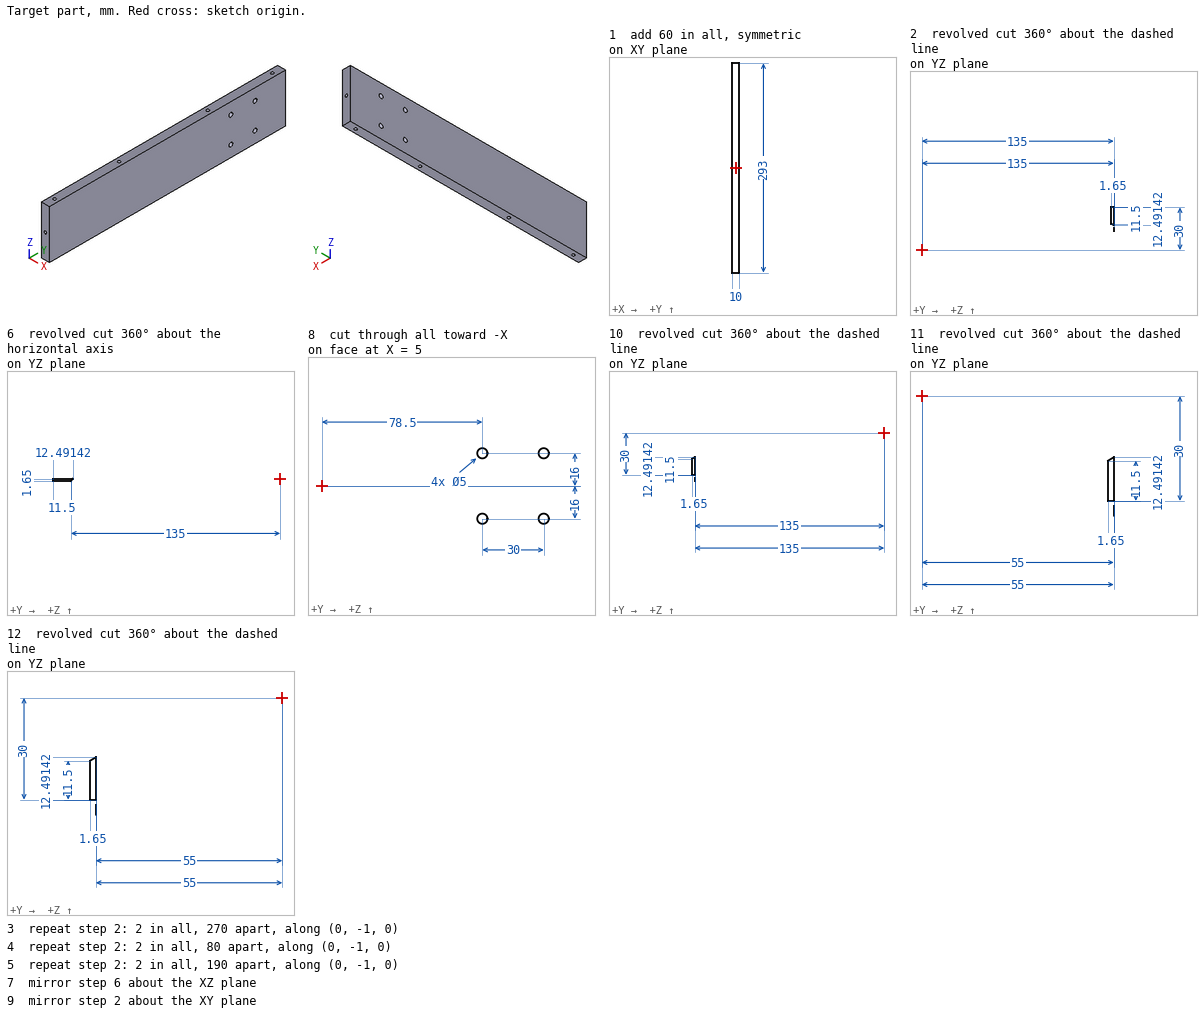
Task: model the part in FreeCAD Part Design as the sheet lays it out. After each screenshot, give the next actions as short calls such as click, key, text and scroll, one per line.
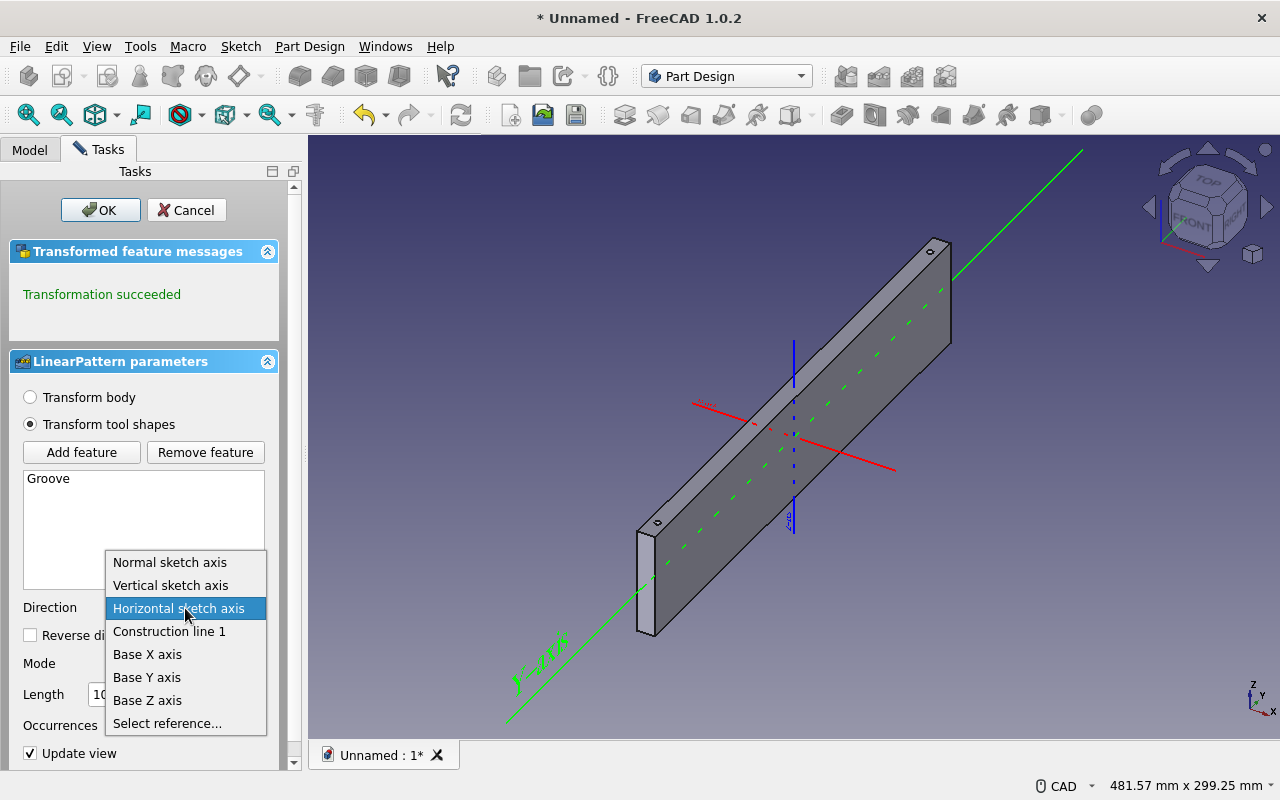
click(184, 678)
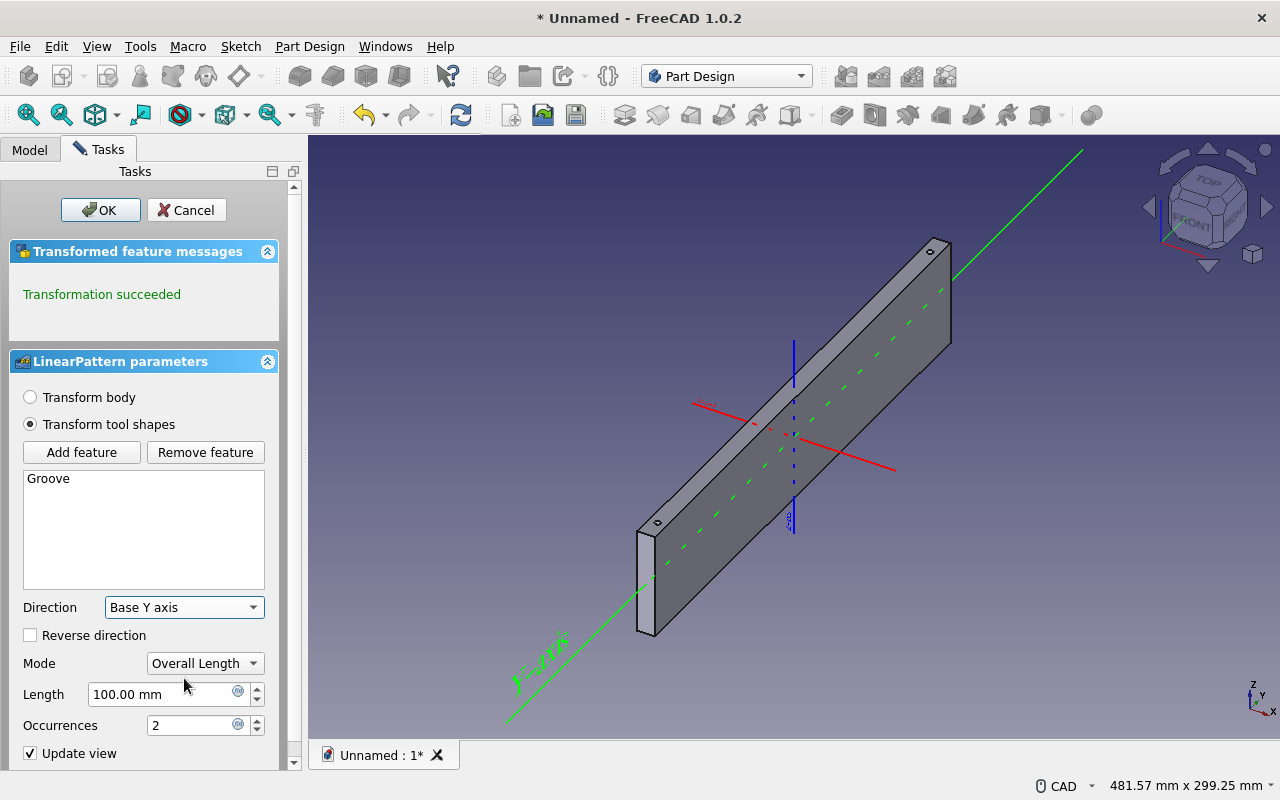
click(206, 664)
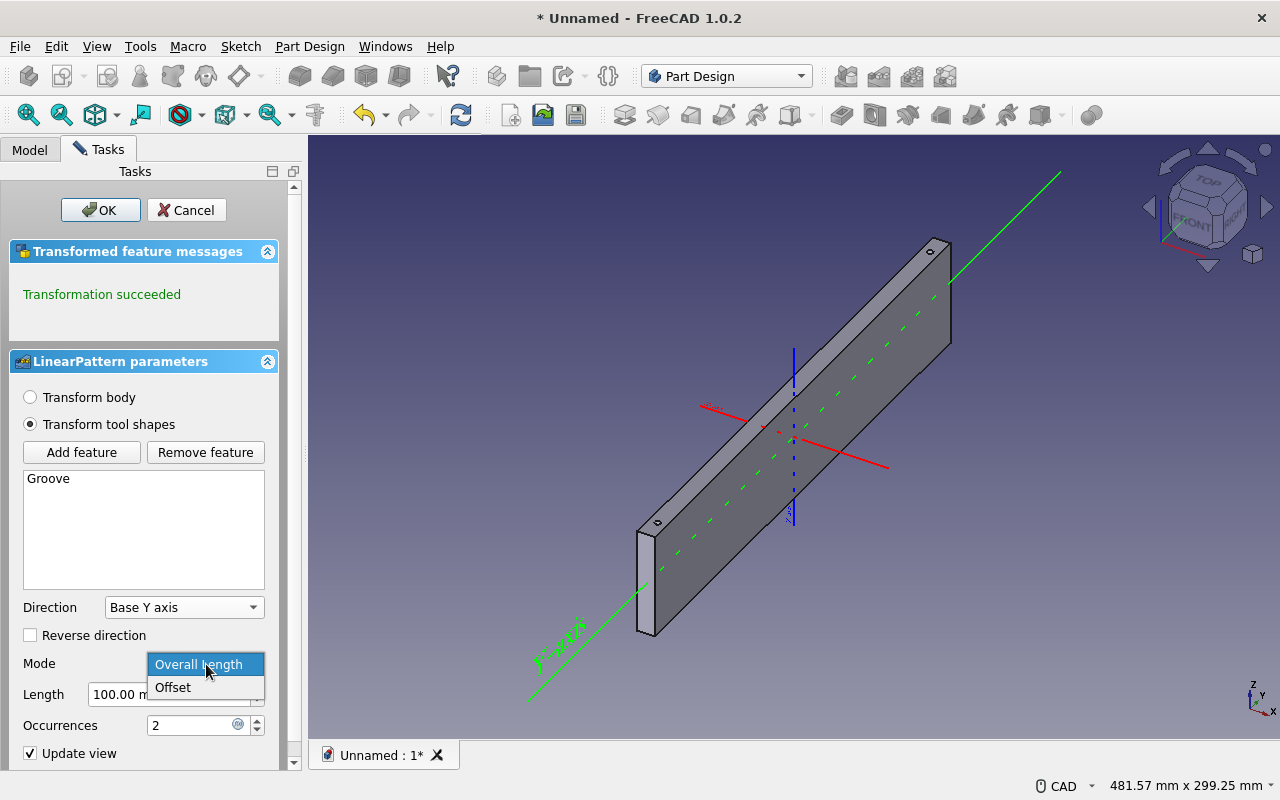
click(204, 688)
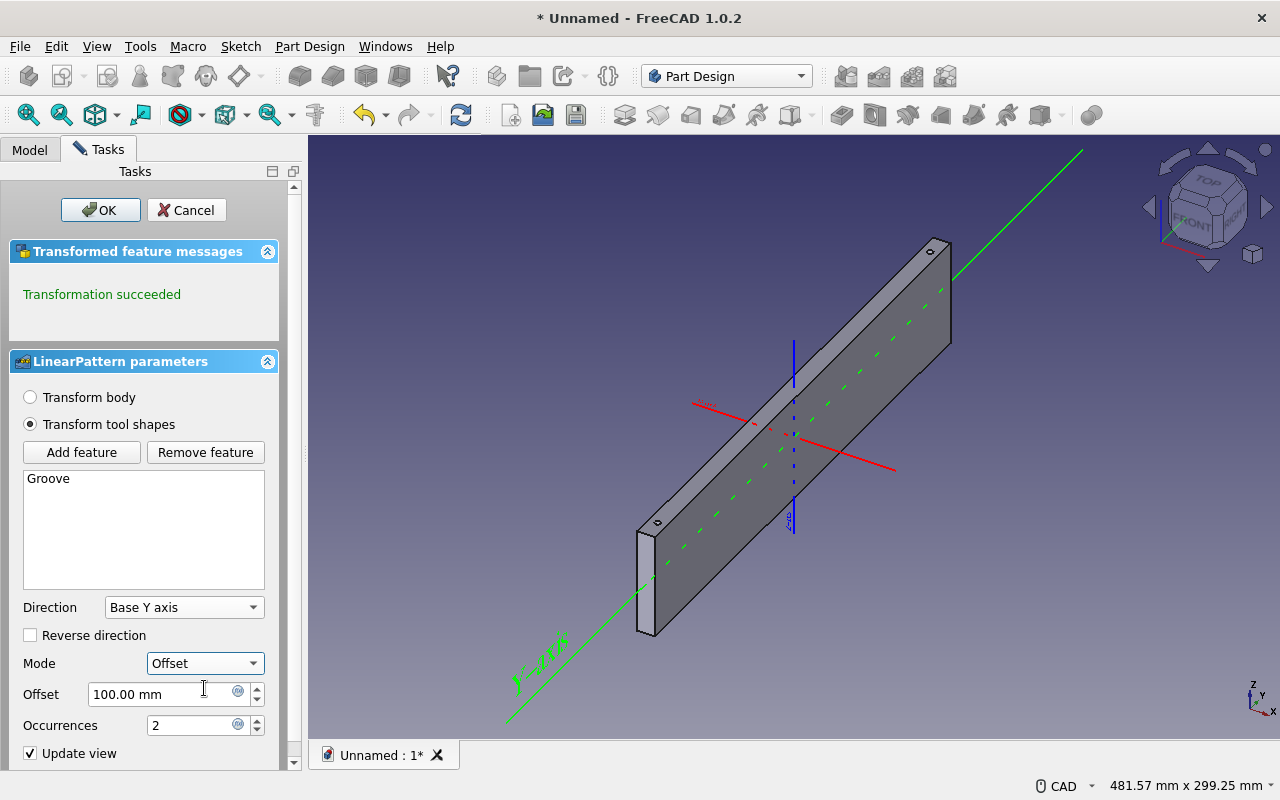
triple_click(170, 694)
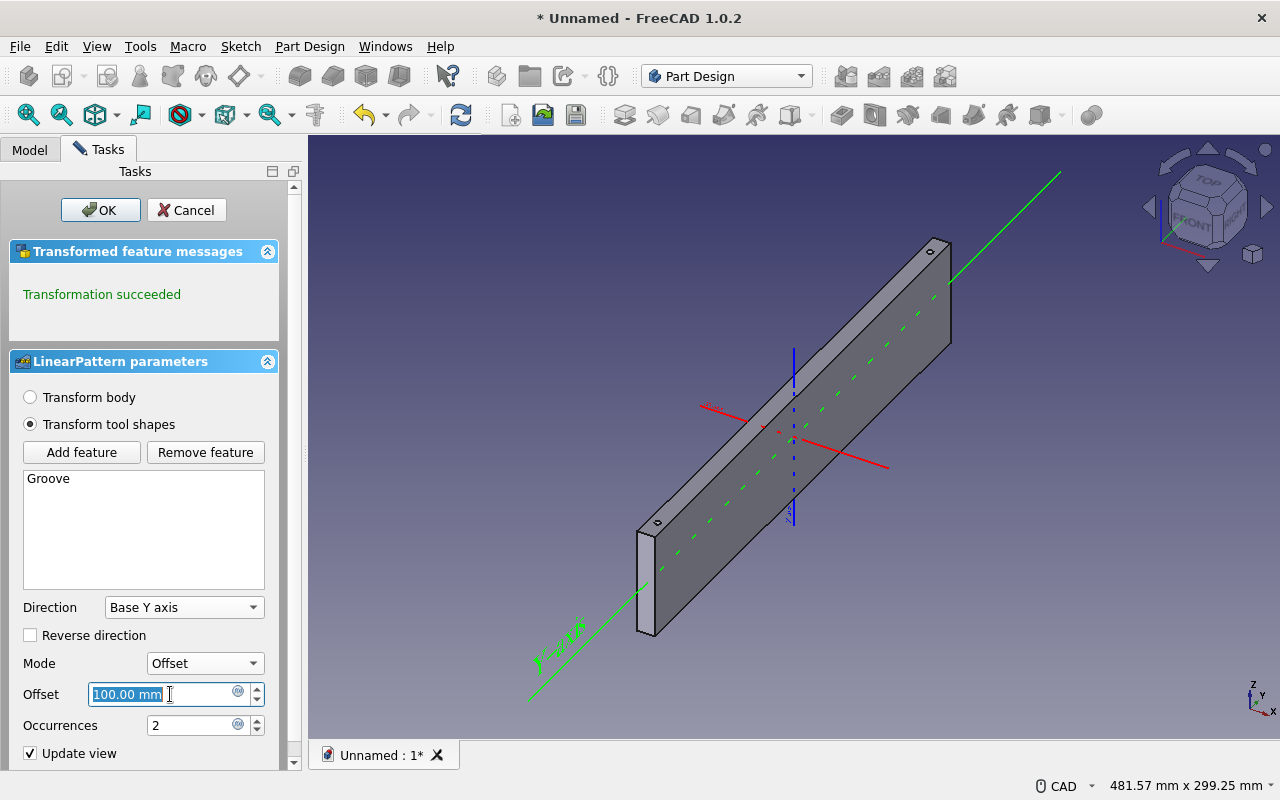
text(80)
key(Tab)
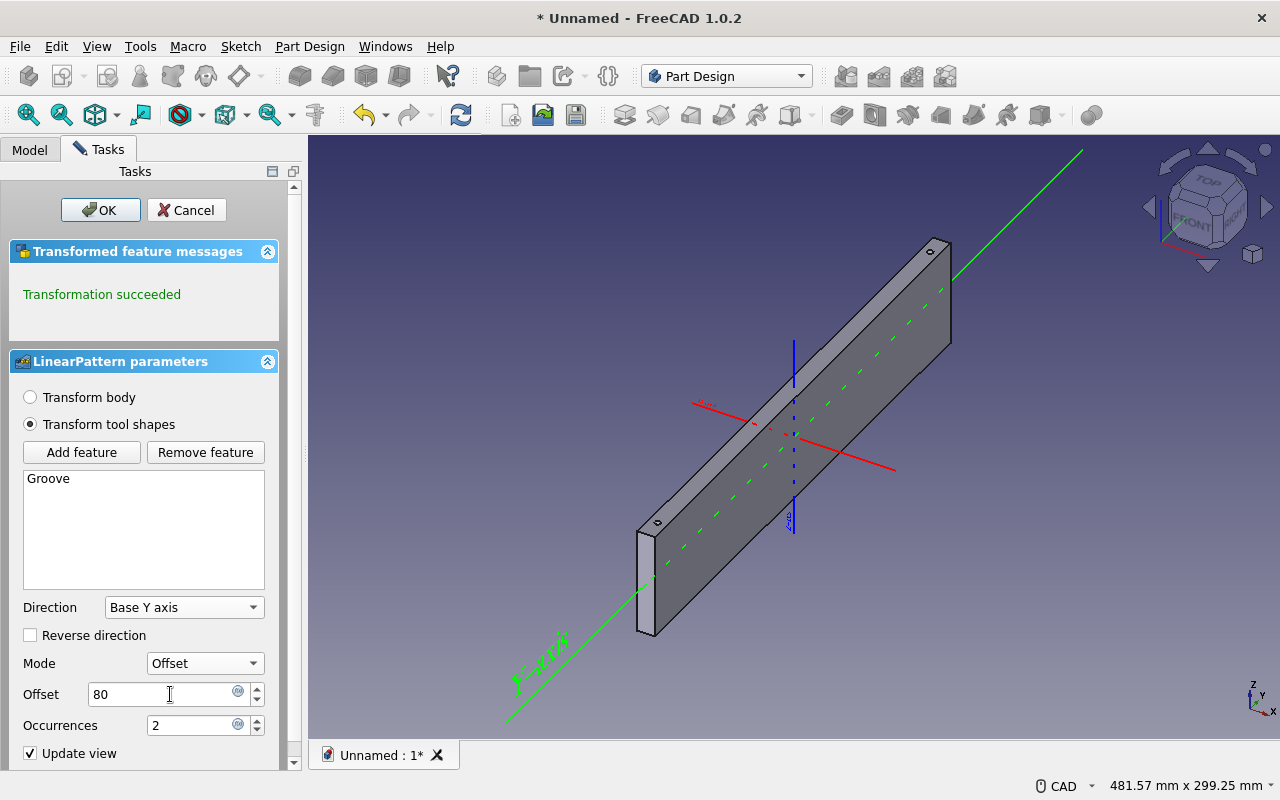
triple_click(199, 726)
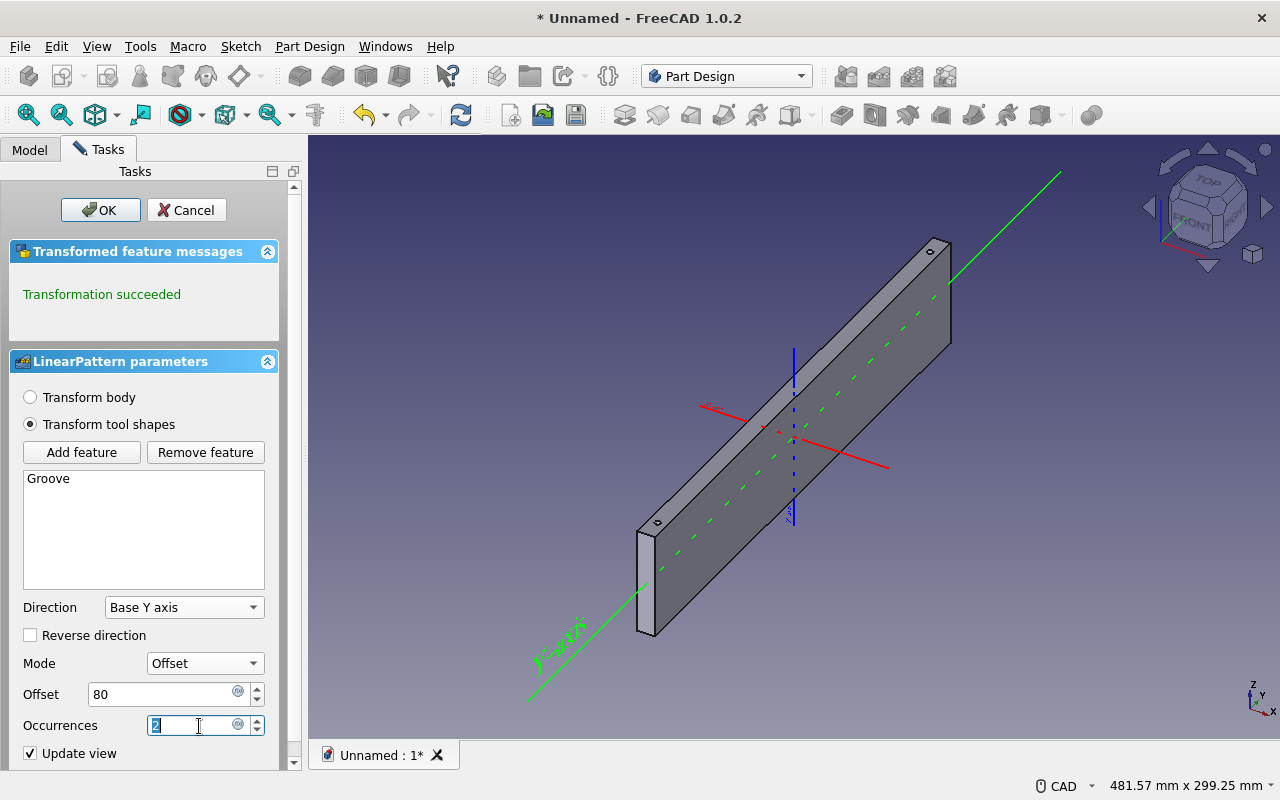
text(2)
key(Tab)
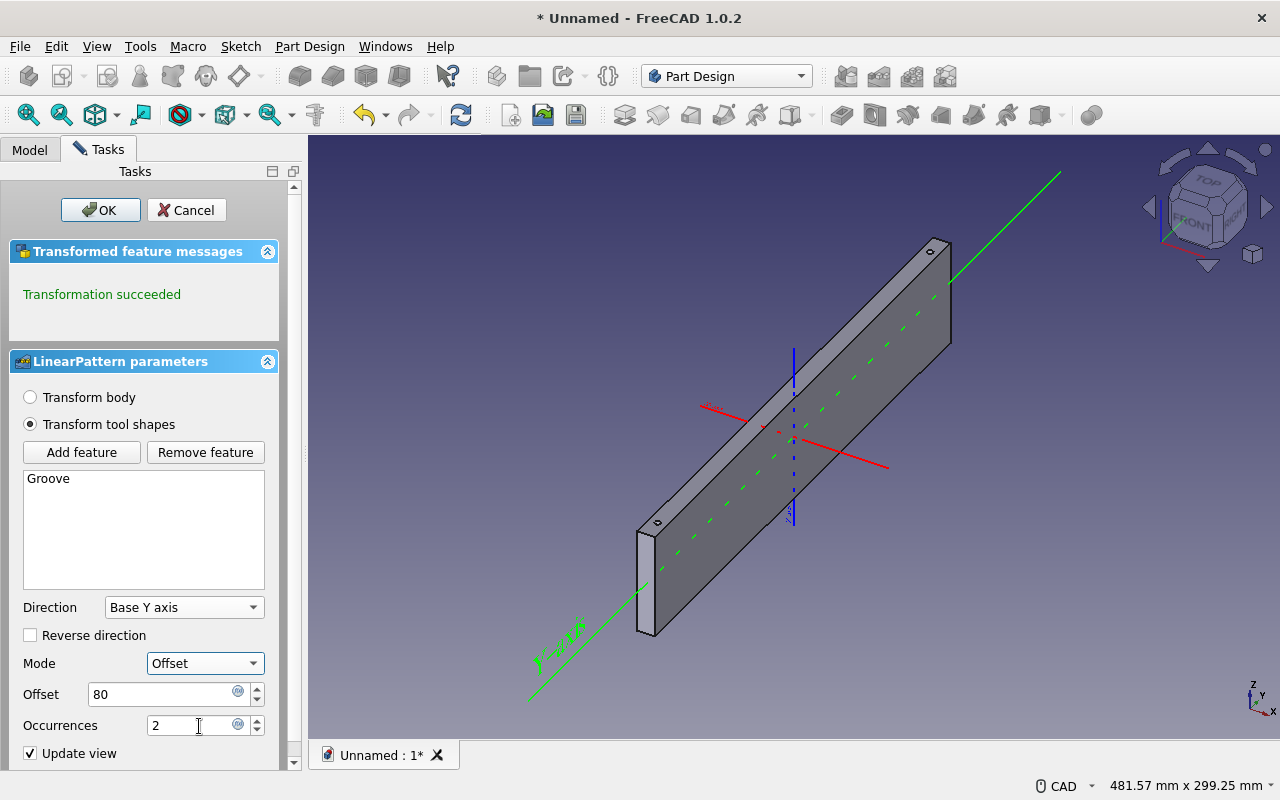
click(31, 635)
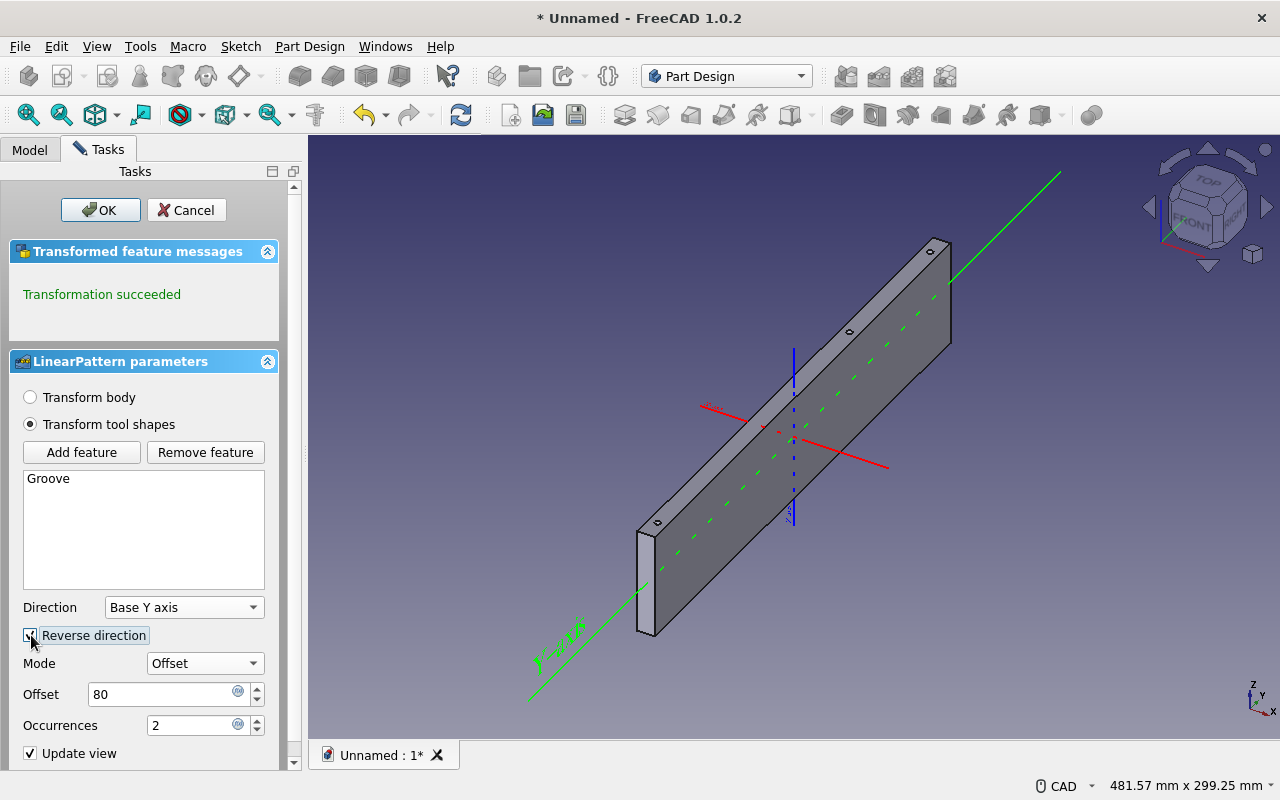
click(101, 210)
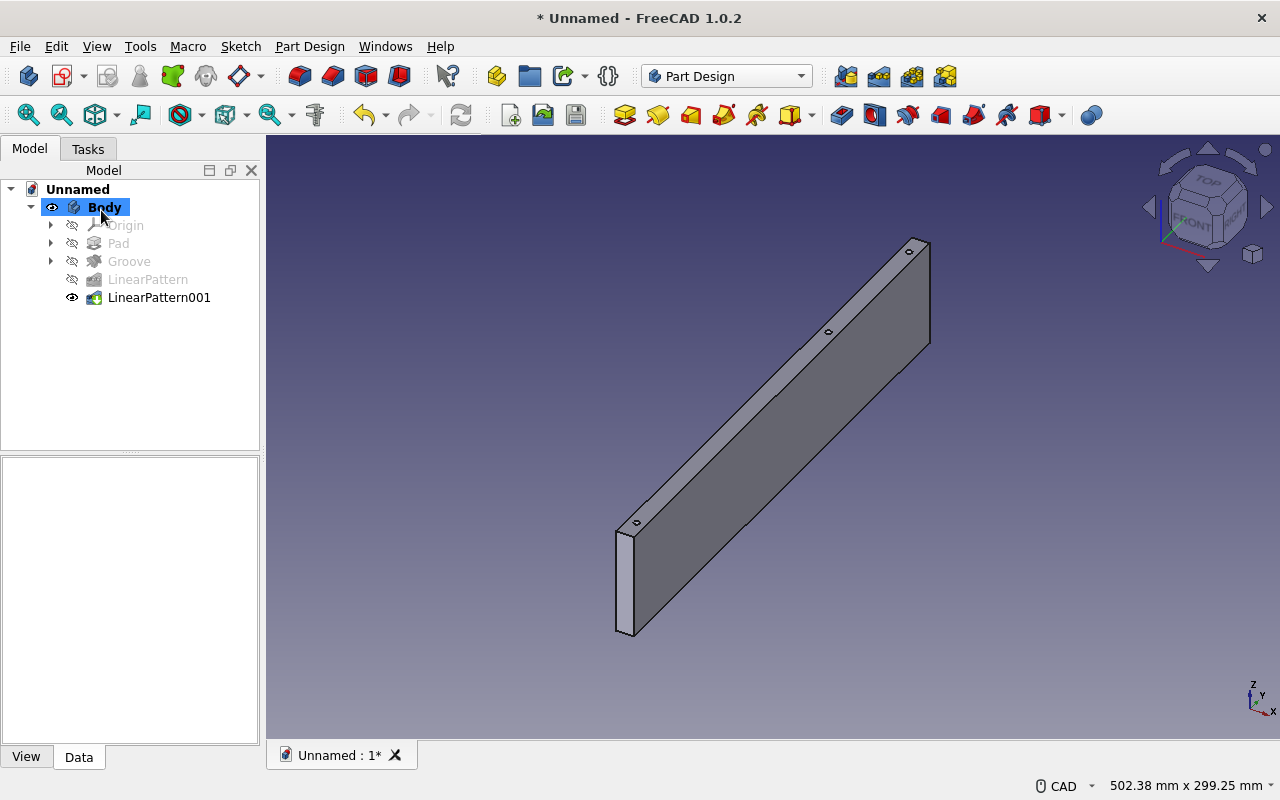
click(117, 261)